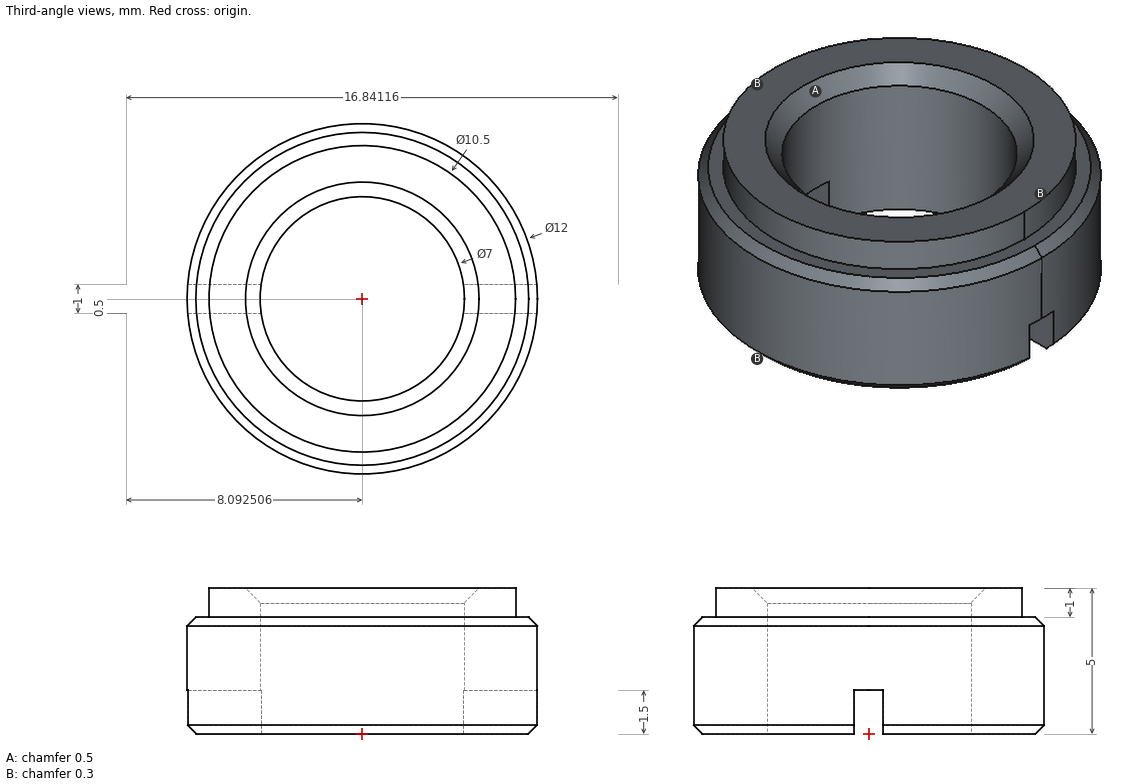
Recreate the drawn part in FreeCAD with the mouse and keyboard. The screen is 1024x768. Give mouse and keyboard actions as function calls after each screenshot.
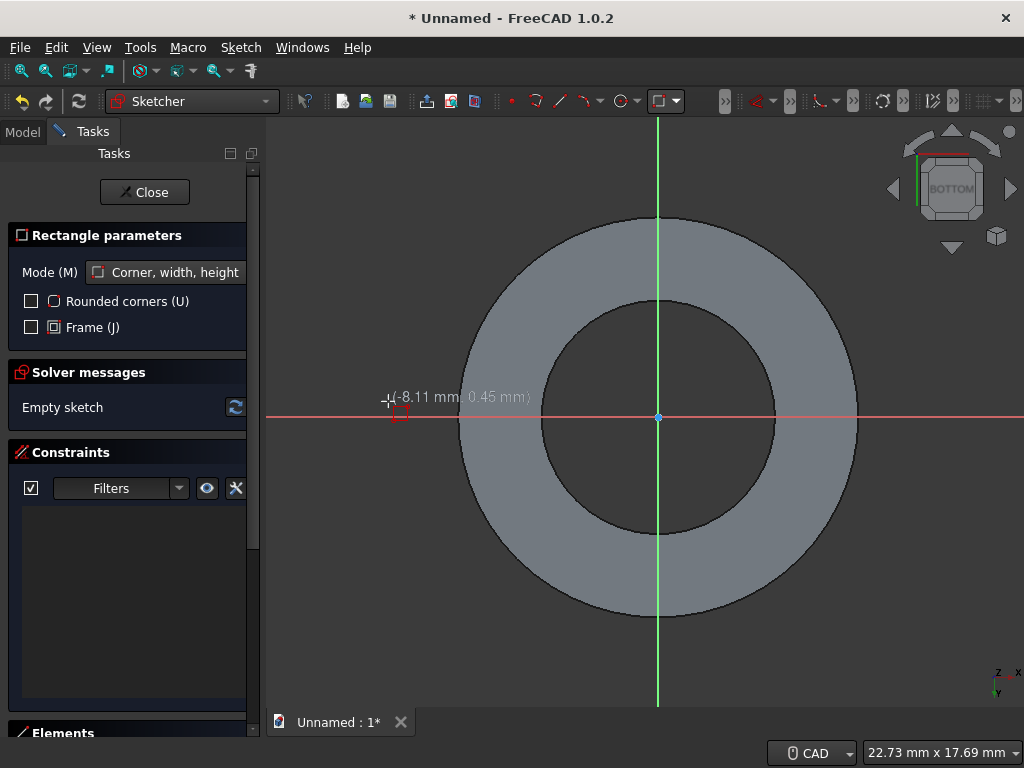
click(388, 401)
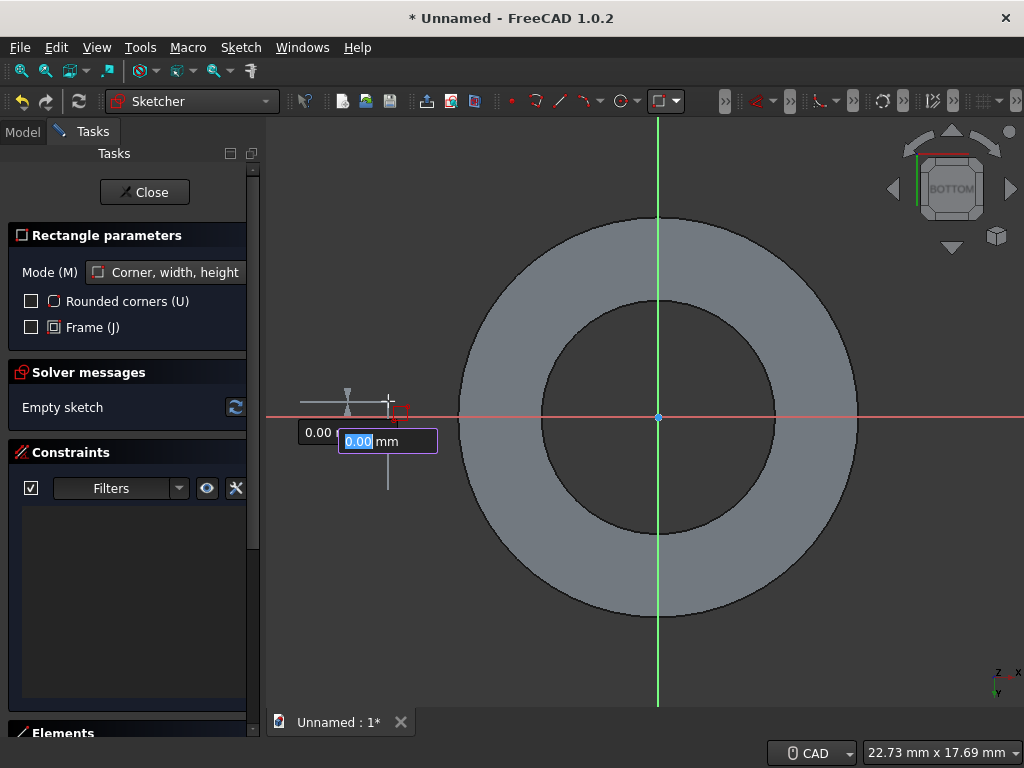
scroll(388, 401, down, 2)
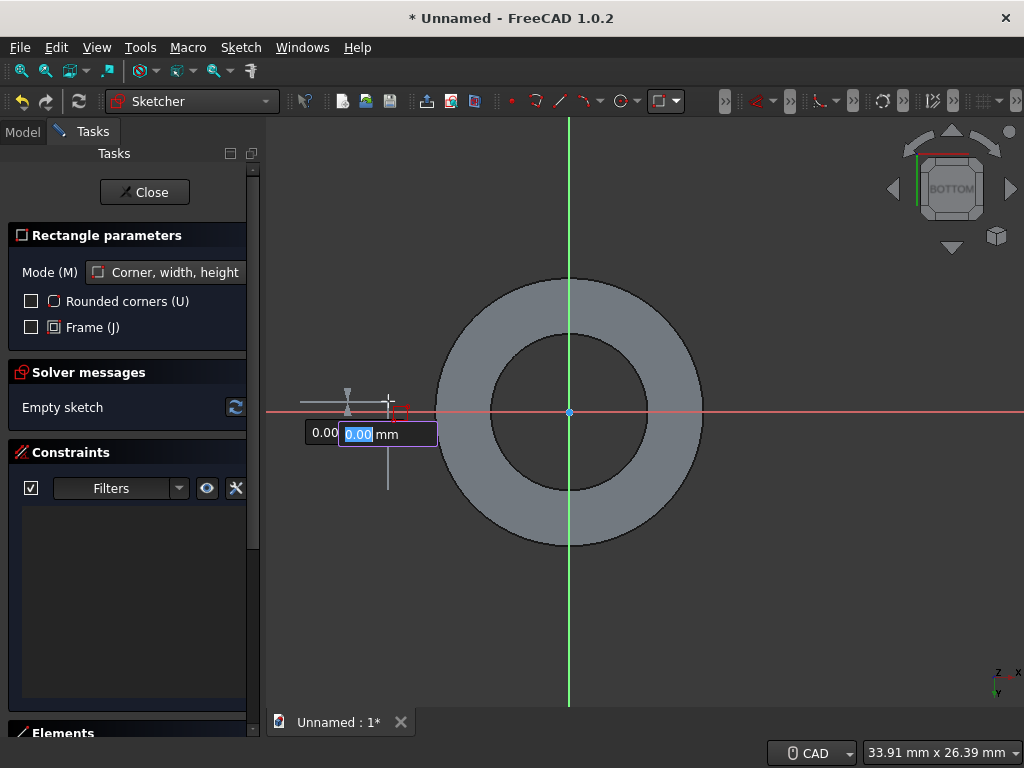
scroll(765, 423, up, 2)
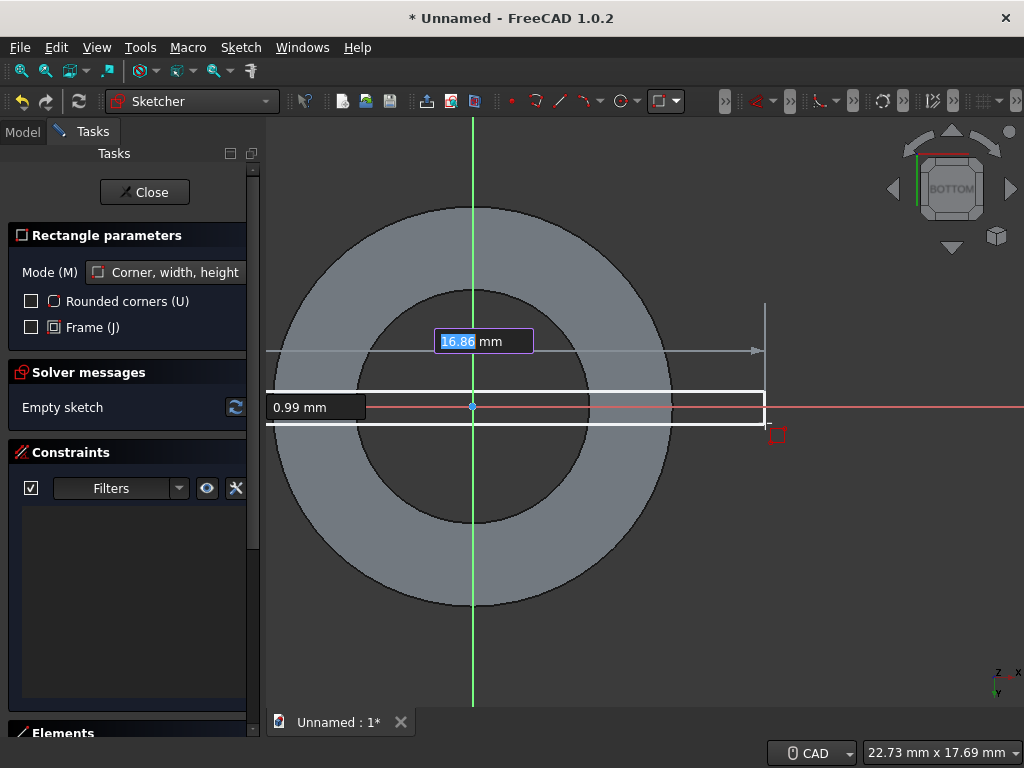
click(764, 423)
key(Escape)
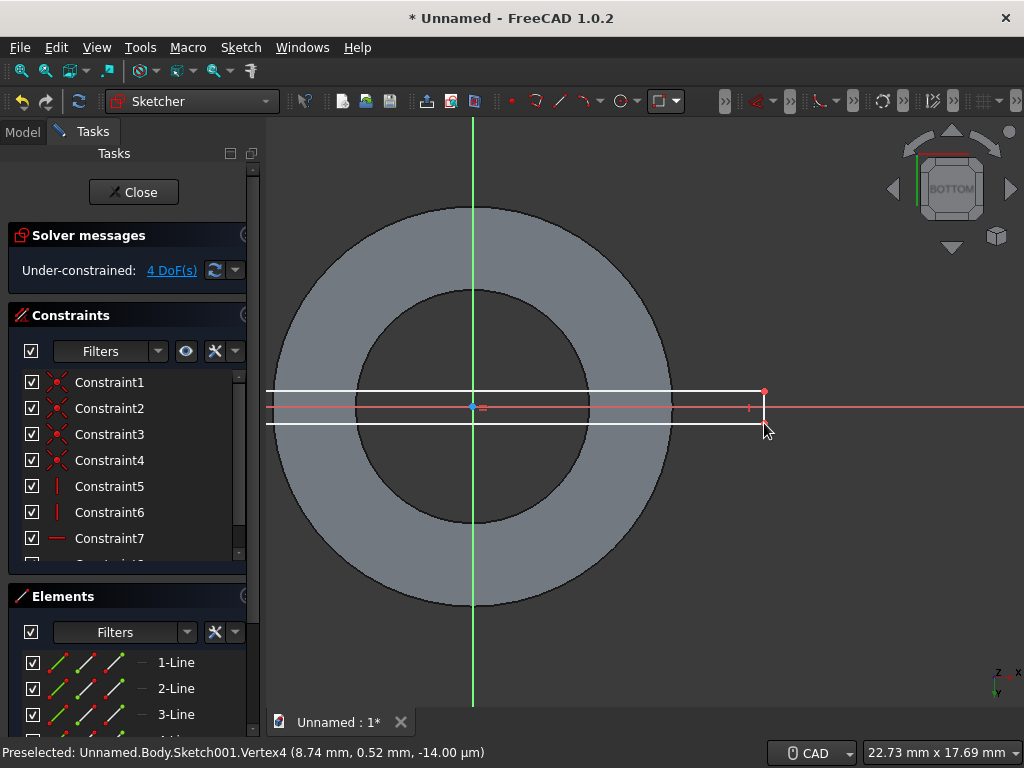
click(756, 102)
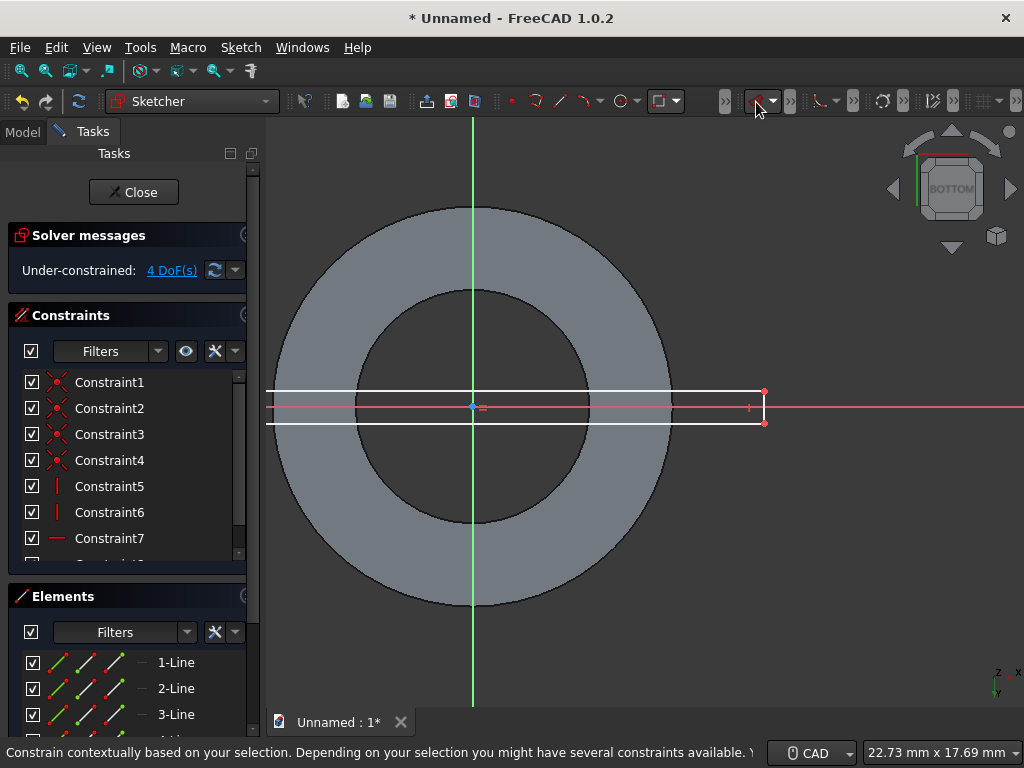
scroll(765, 423, down, 2)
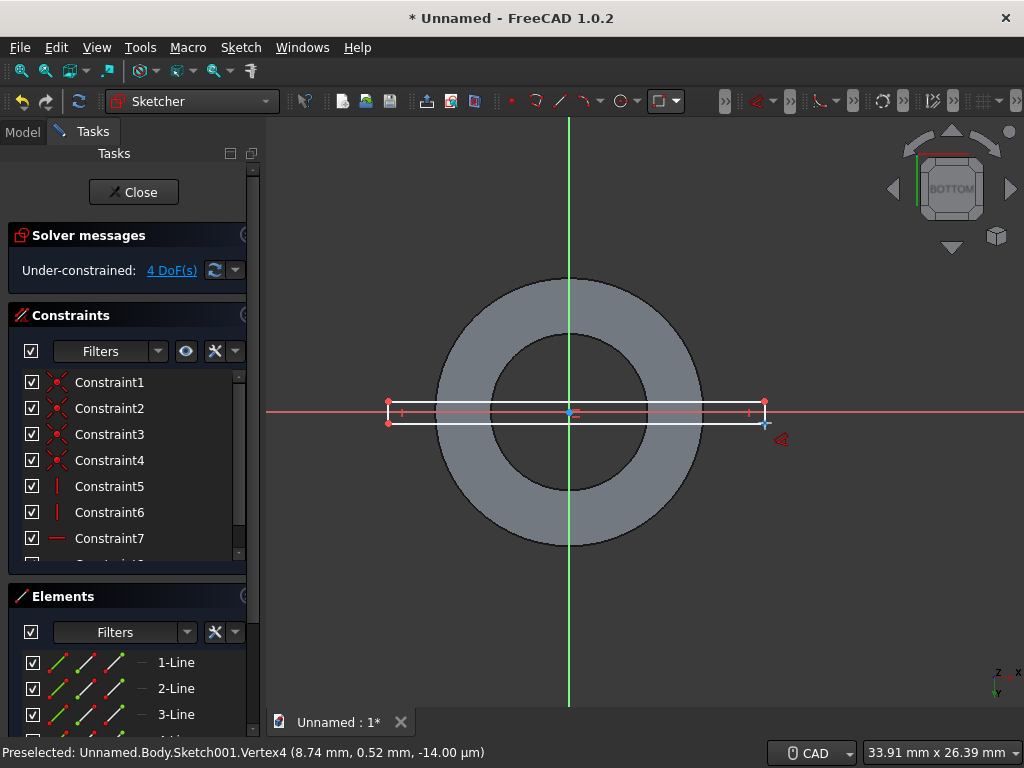
scroll(388, 411, up, 3)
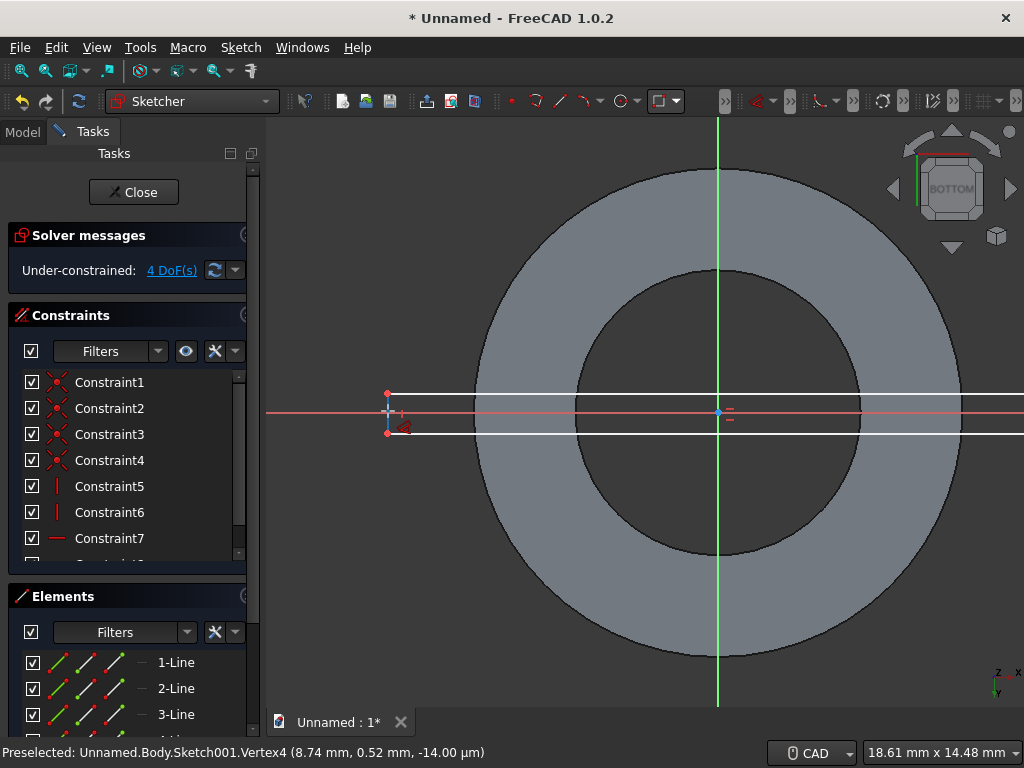
click(388, 410)
click(354, 428)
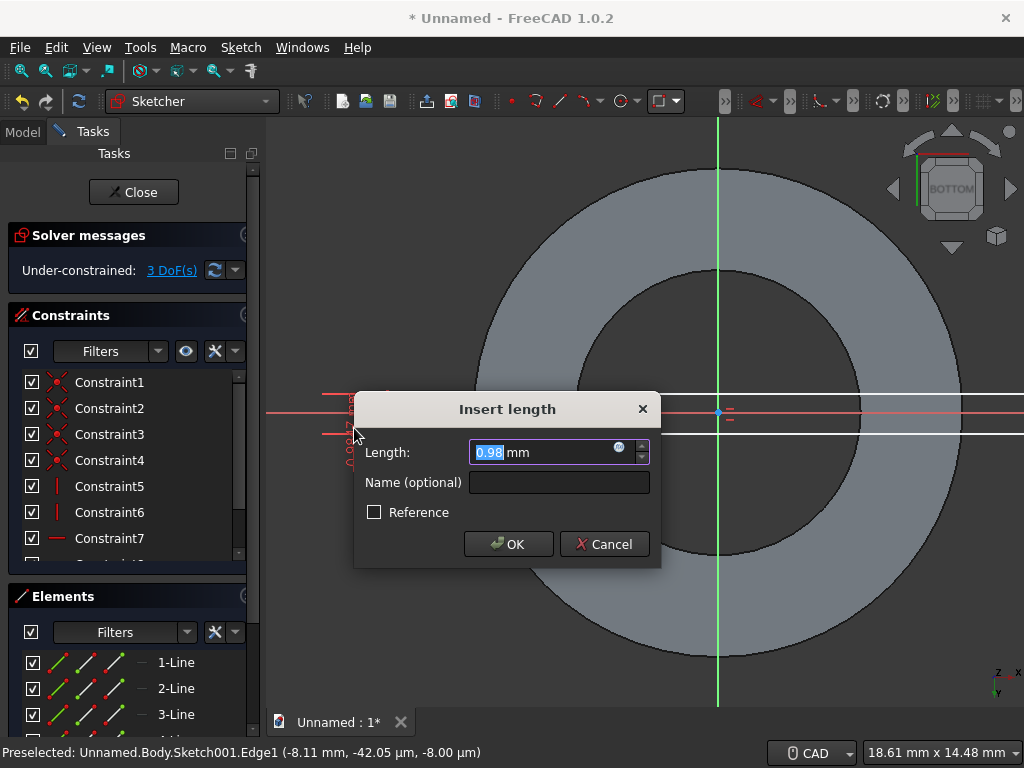
text(1)
key(Return)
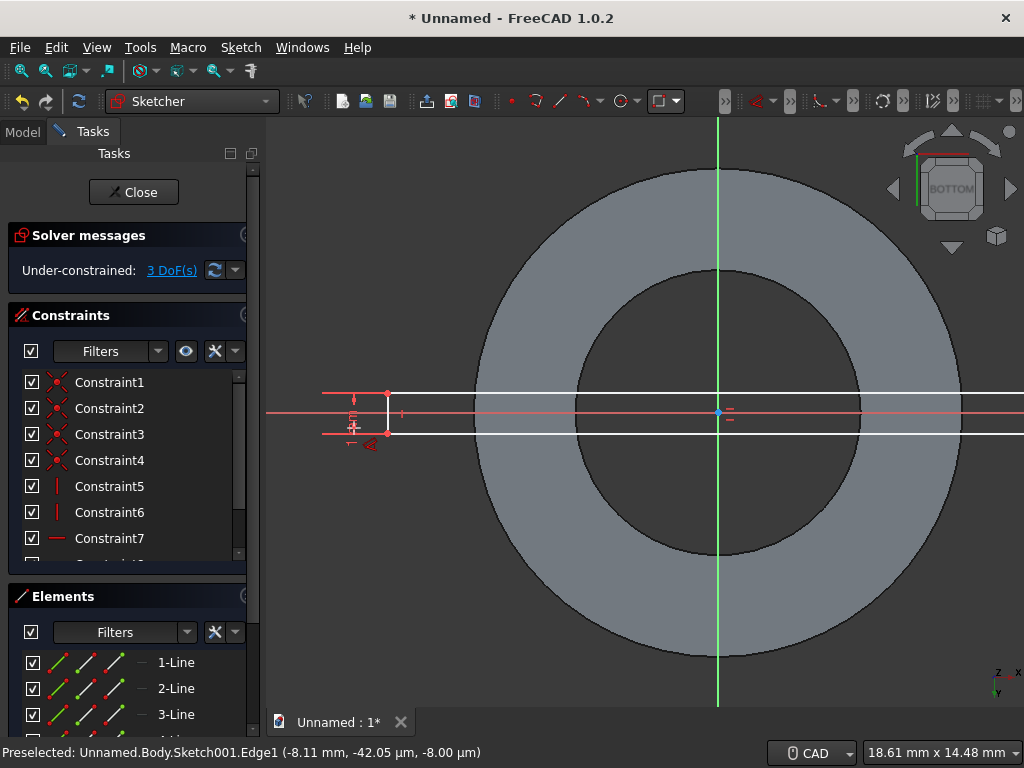
scroll(388, 393, up, 4)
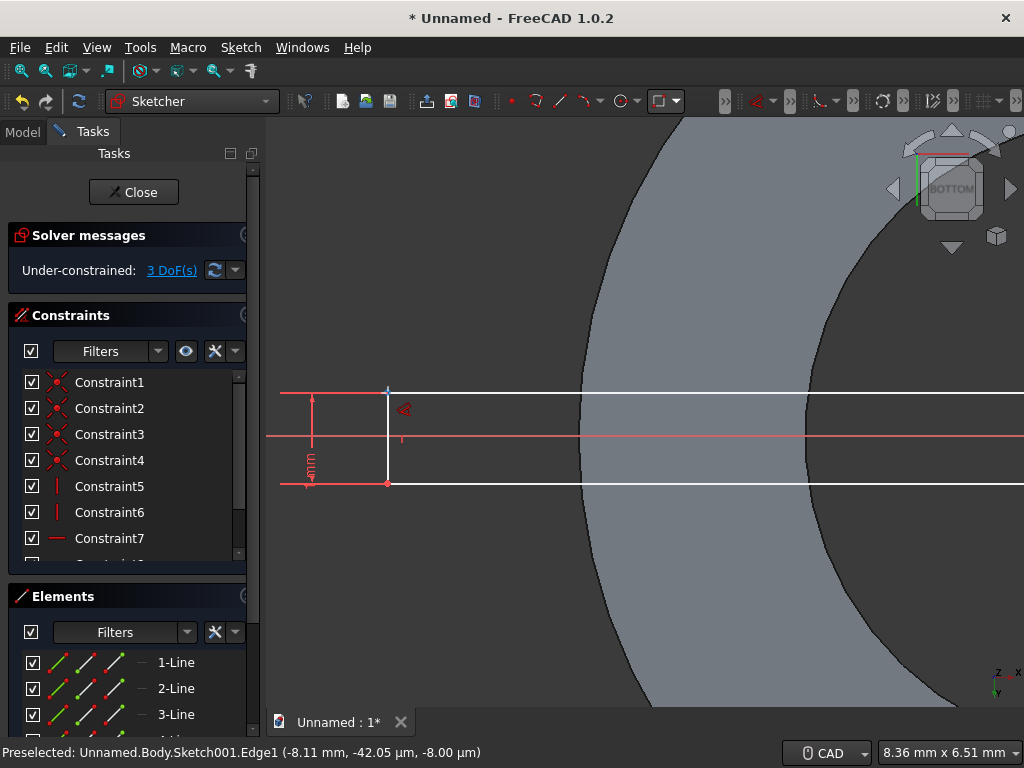
click(388, 393)
click(354, 415)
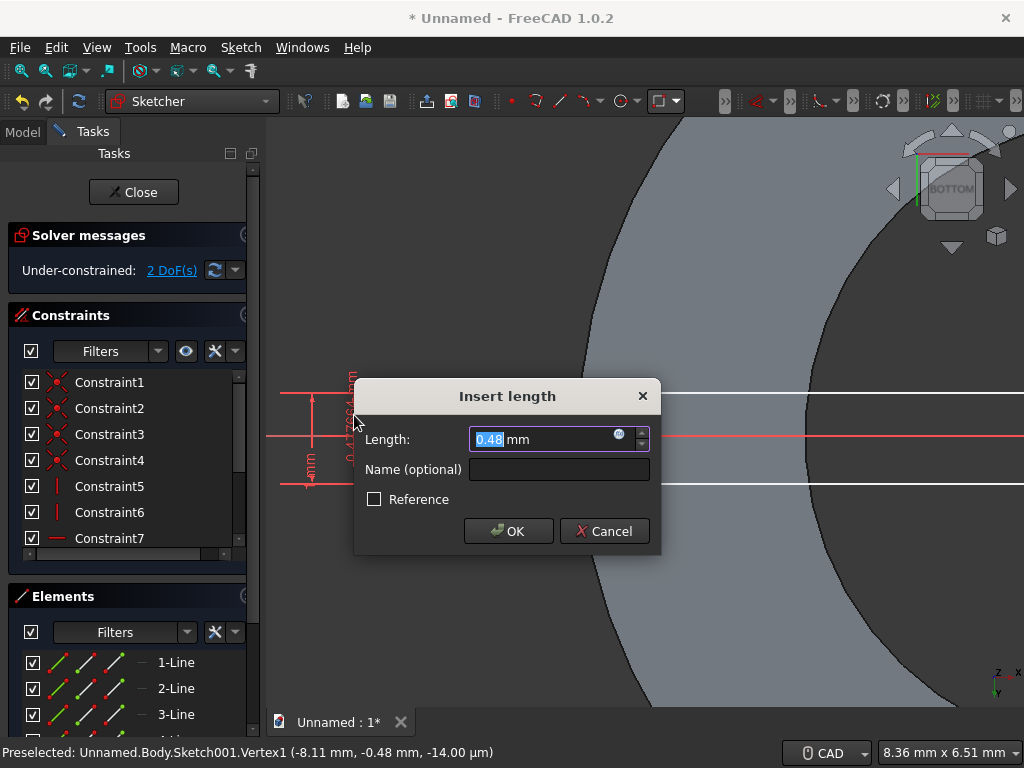
text(0.5)
key(Return)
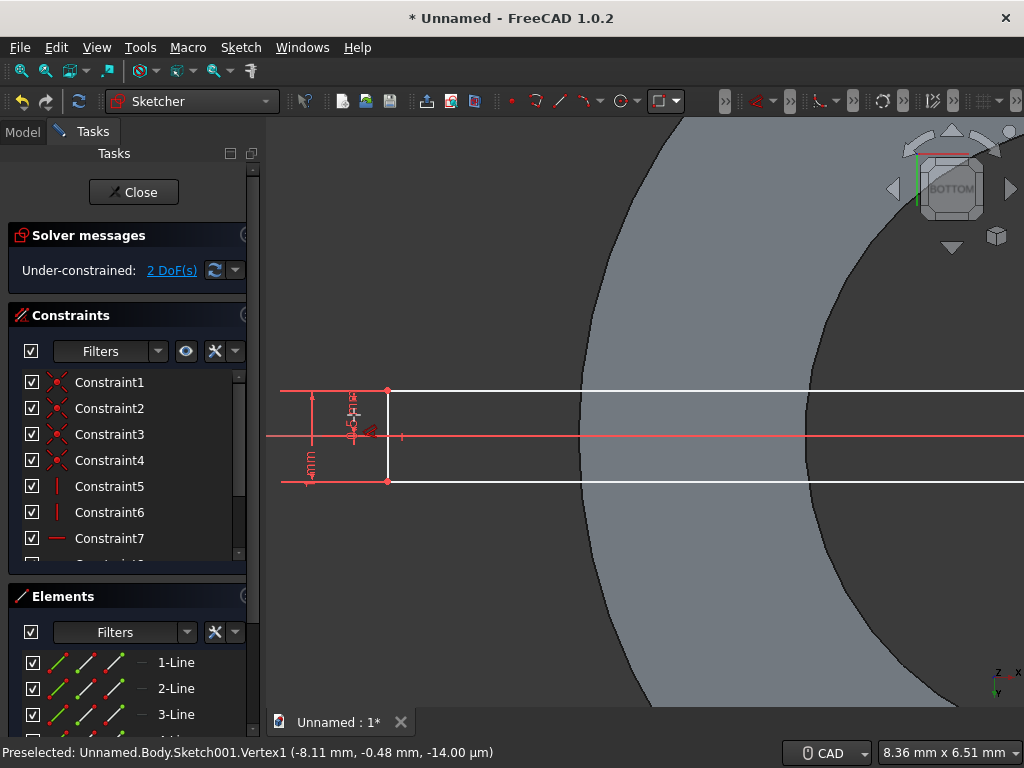
scroll(388, 404, down, 7)